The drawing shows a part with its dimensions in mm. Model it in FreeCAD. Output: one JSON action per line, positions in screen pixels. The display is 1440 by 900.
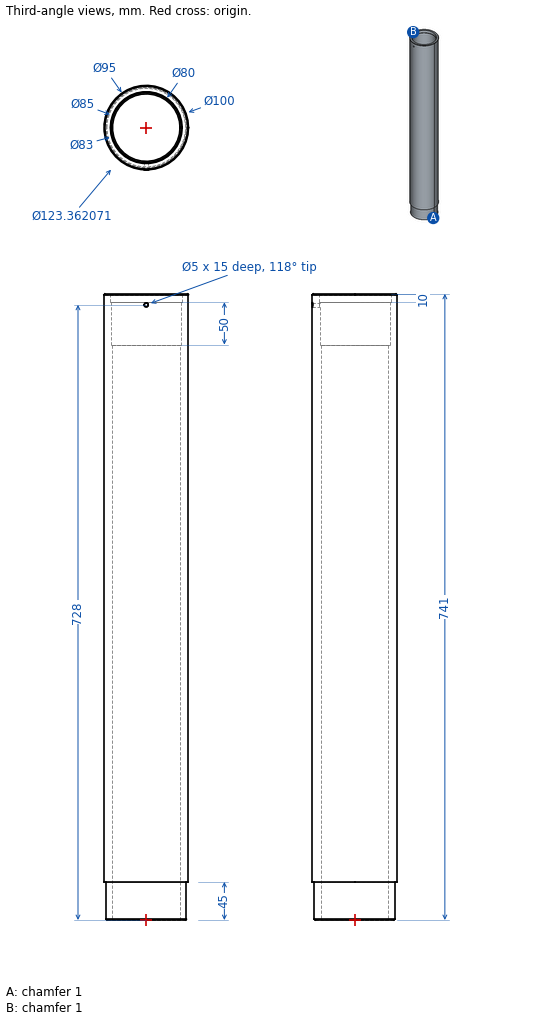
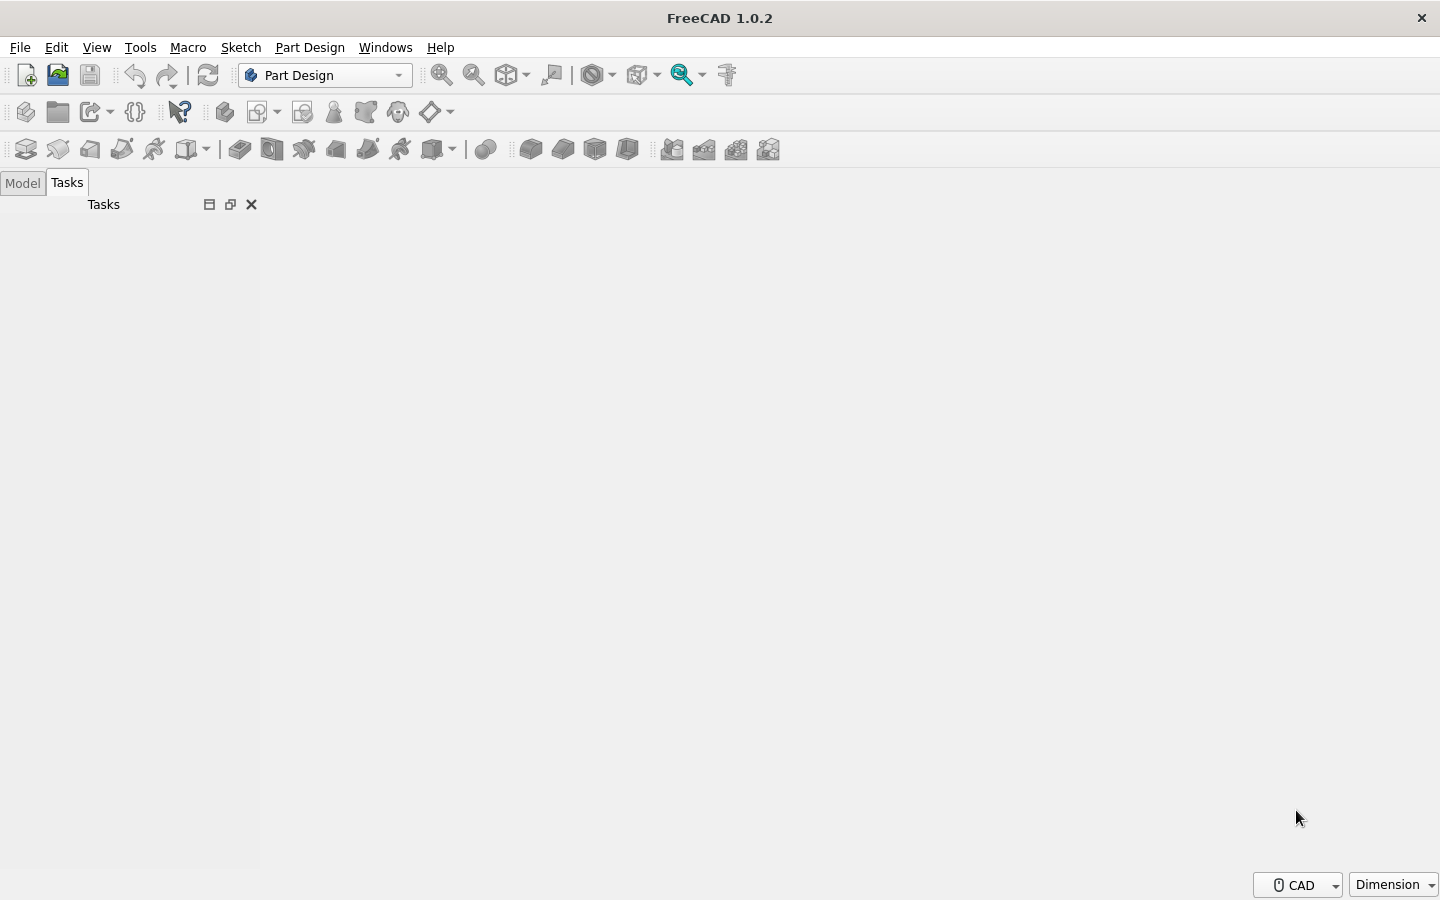
{"action": "left_click", "coordinate": [26, 76]}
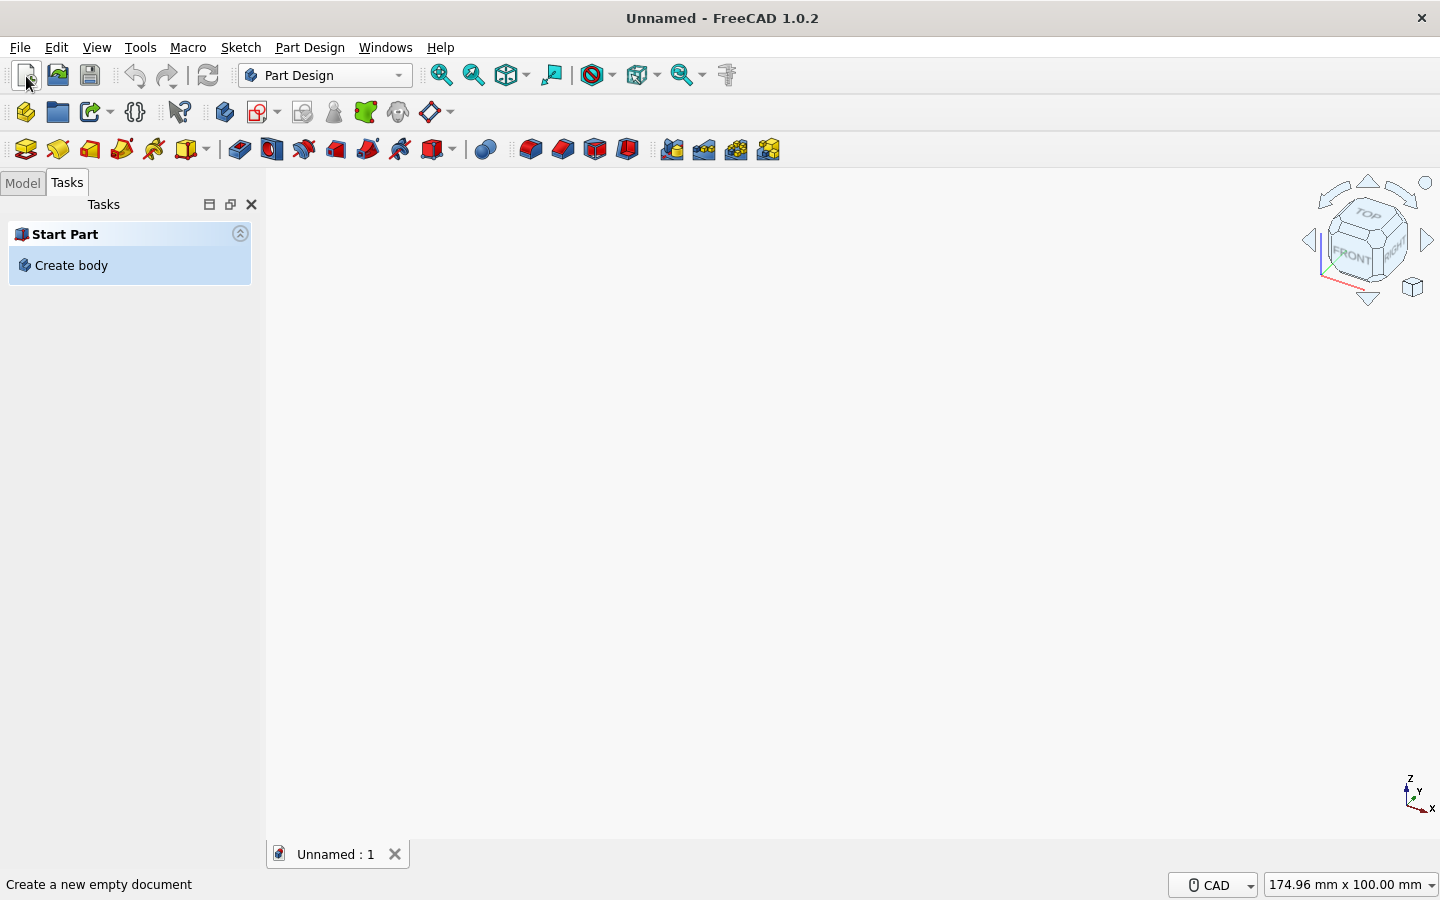
{"action": "left_click", "coordinate": [258, 112]}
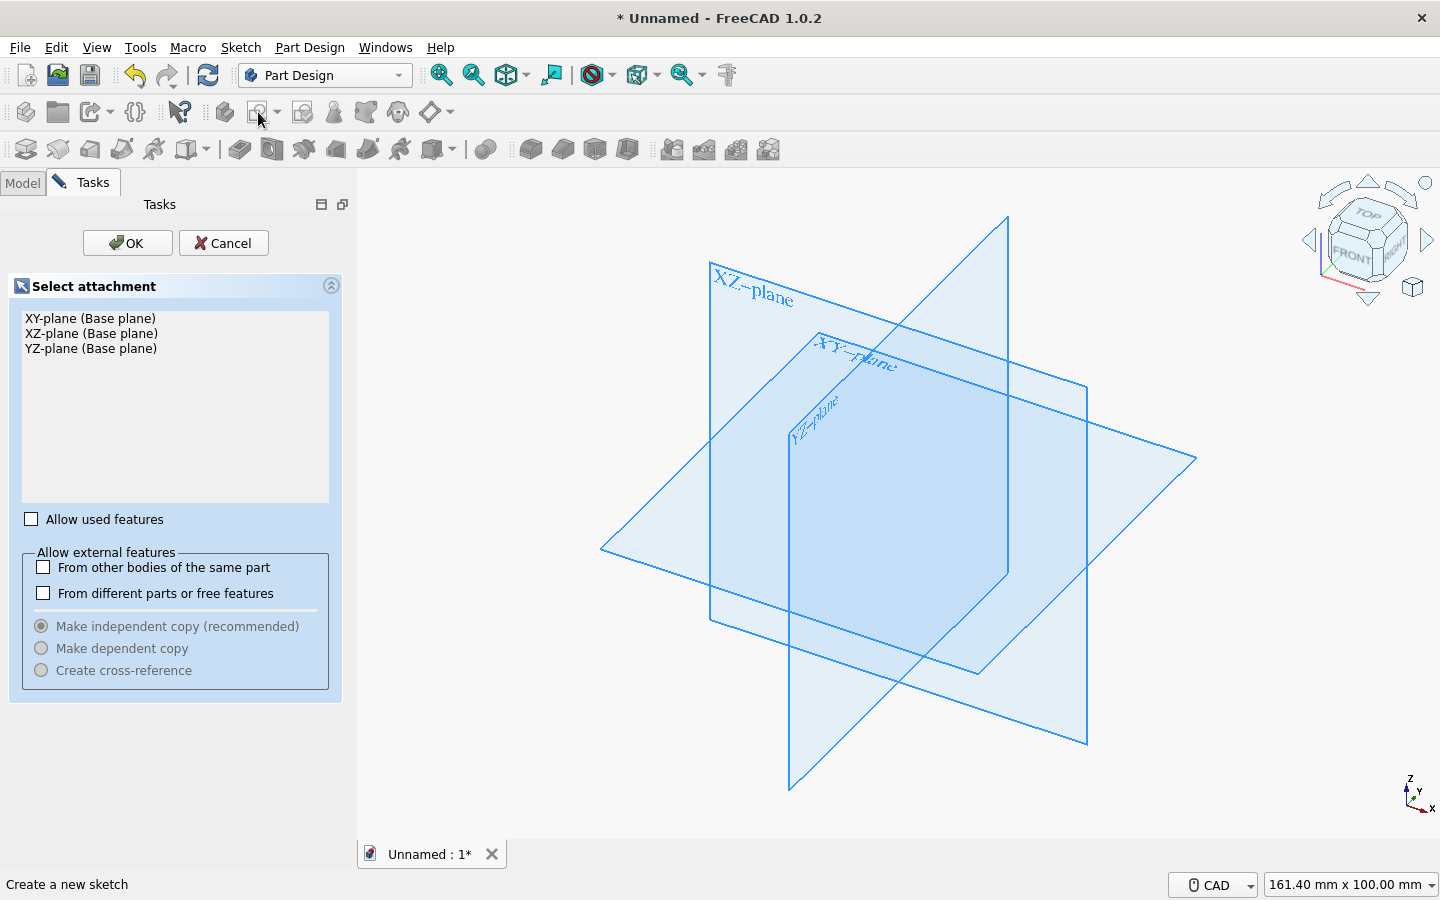
{"action": "left_click", "coordinate": [82, 318]}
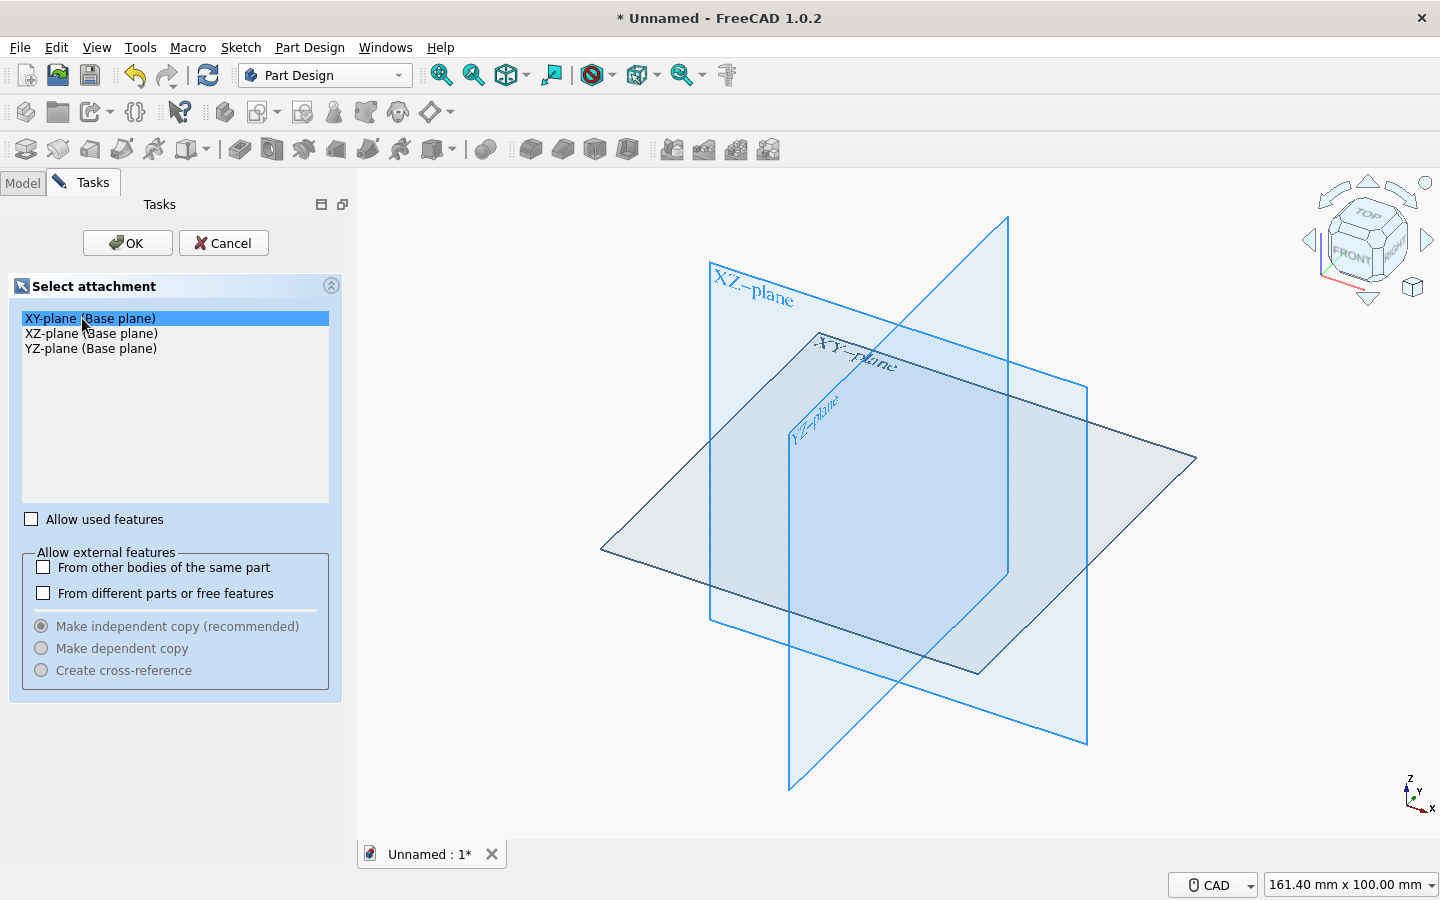
{"action": "left_click", "coordinate": [128, 243]}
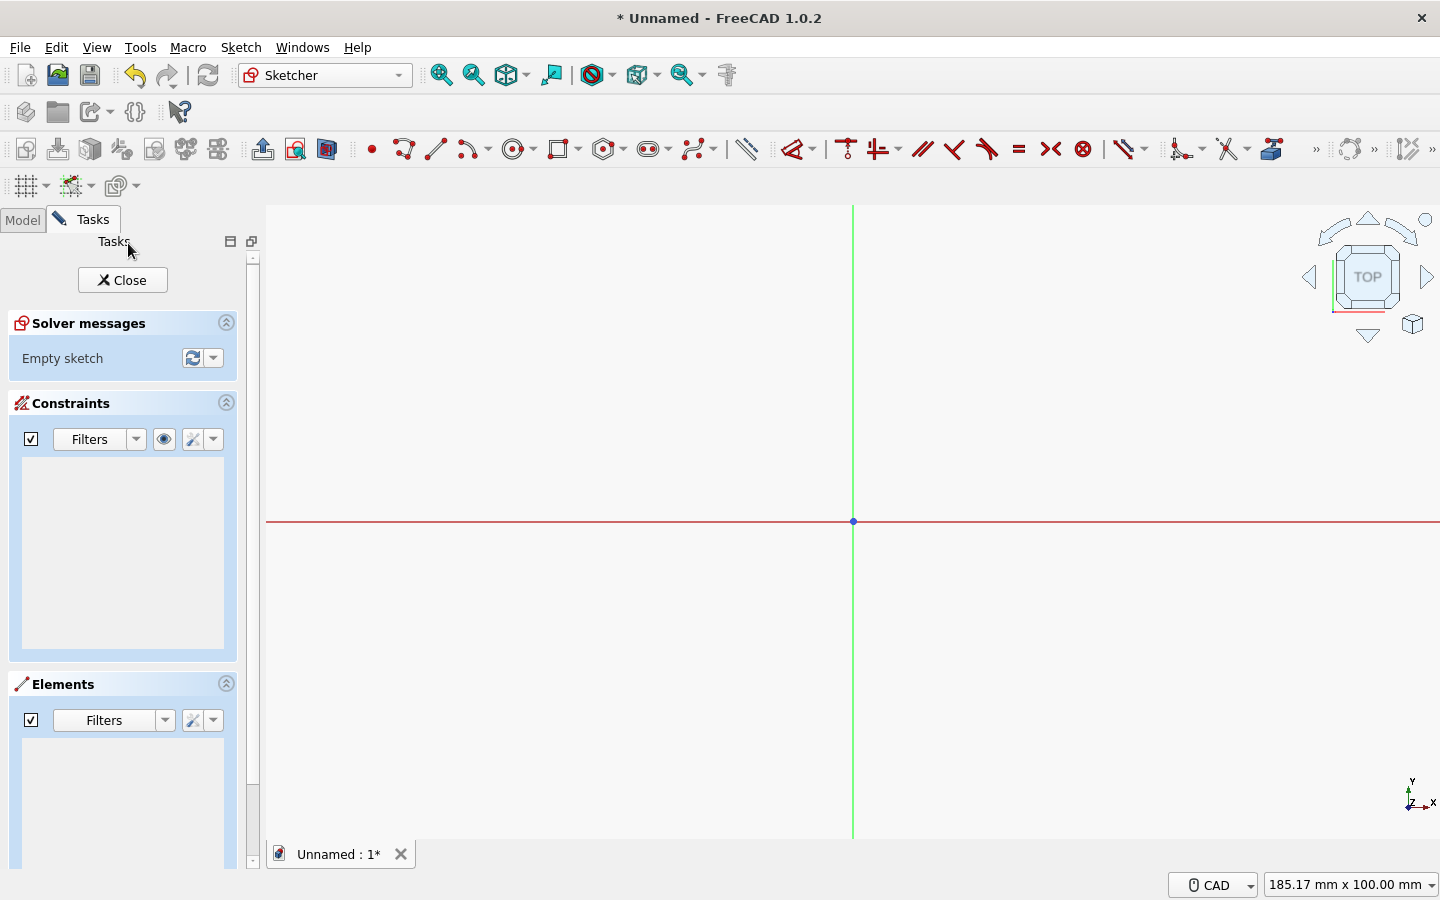
{"action": "scroll", "coordinate": [645, 522], "scroll_direction": "down", "scroll_amount": 2}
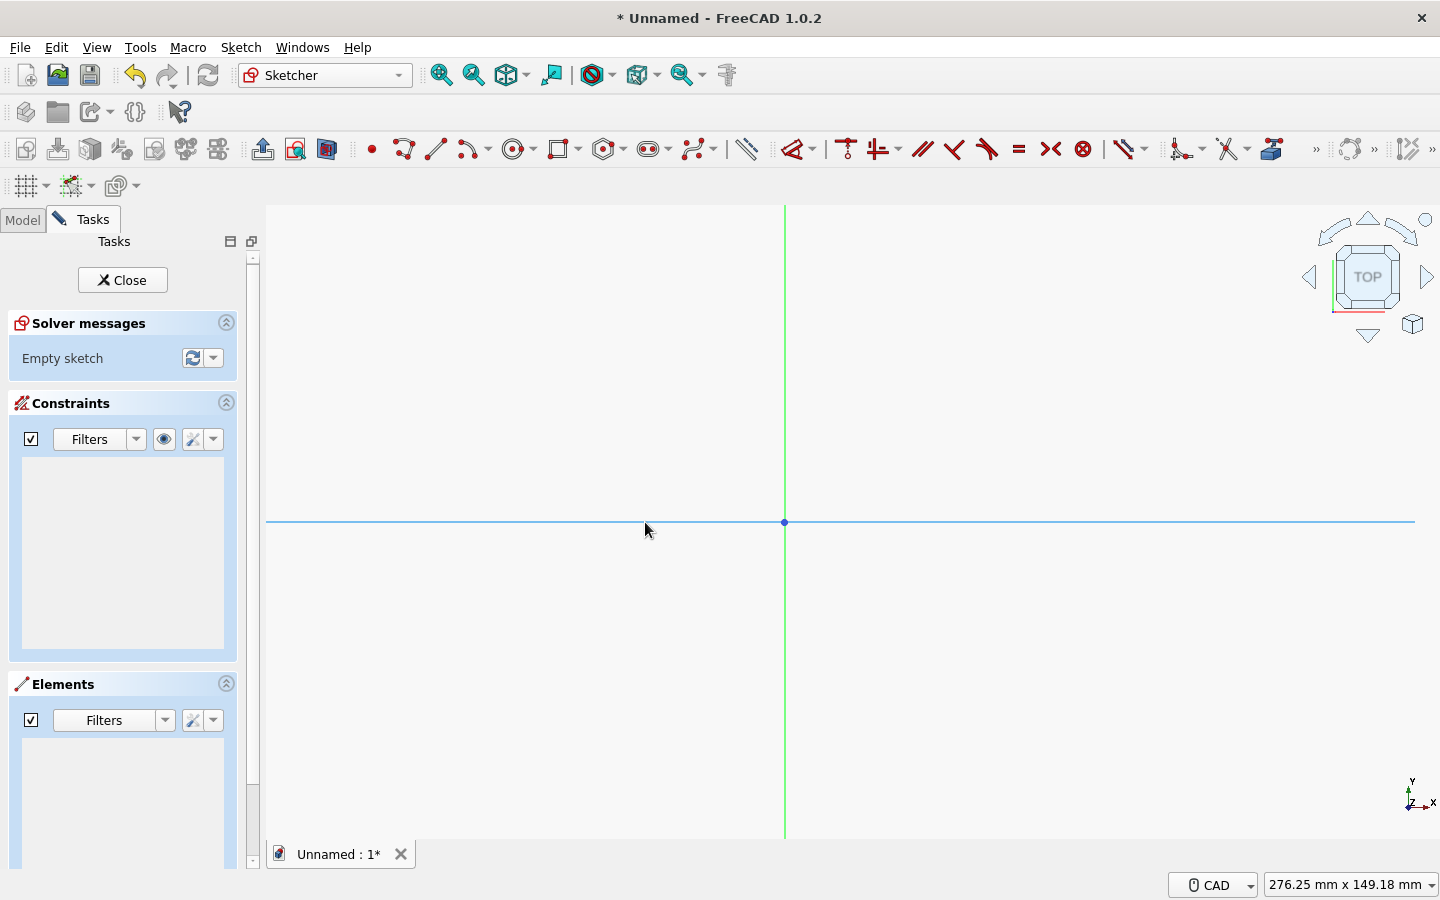
{"action": "left_click", "coordinate": [514, 150]}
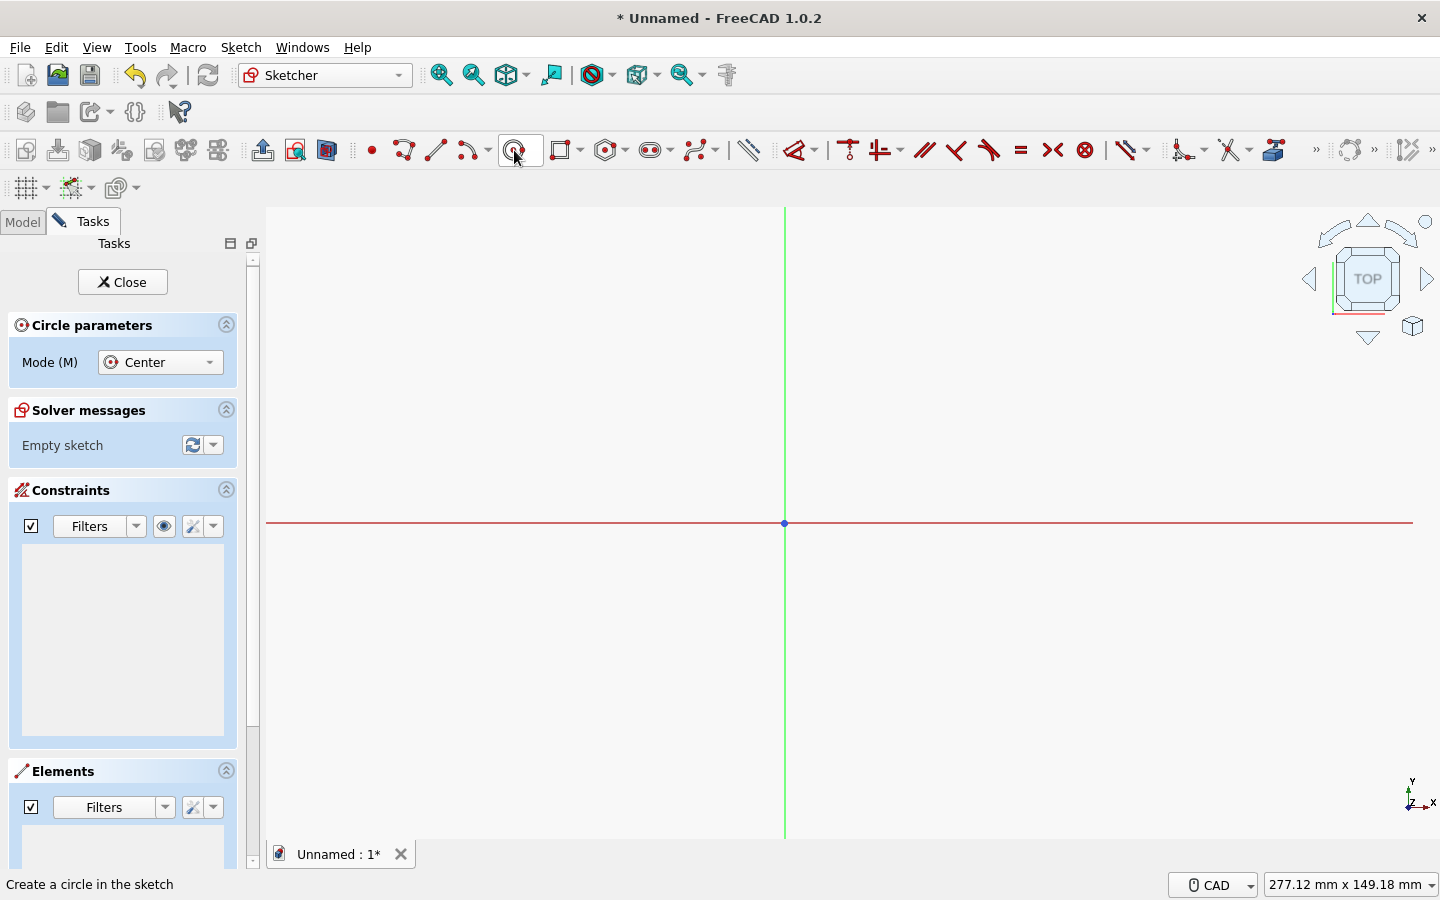
{"action": "left_click", "coordinate": [785, 523]}
{"action": "left_click", "coordinate": [935, 373]}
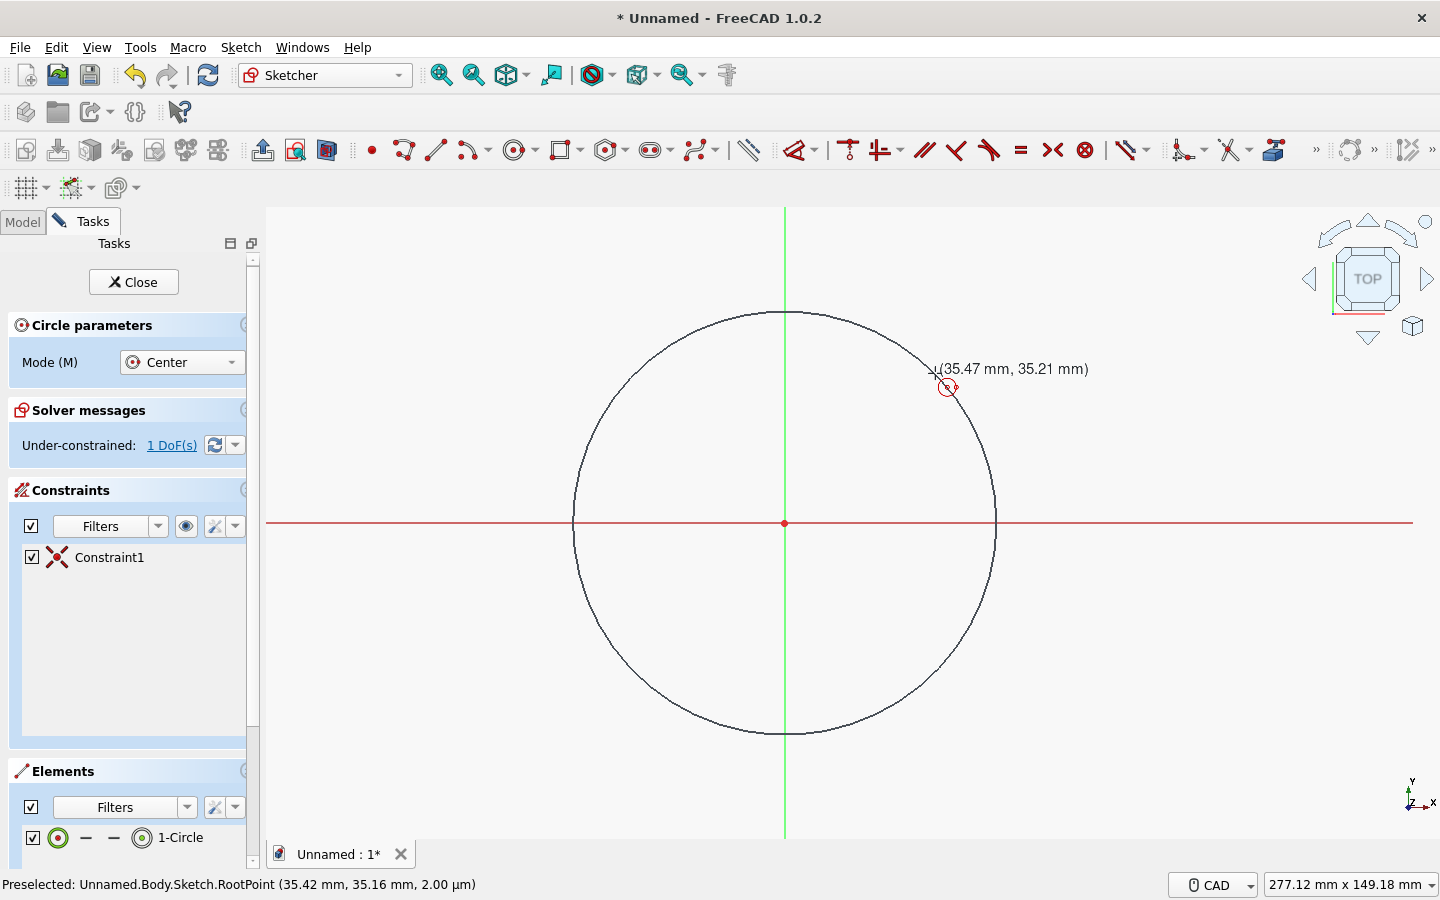
{"action": "left_click", "coordinate": [785, 523]}
{"action": "left_click", "coordinate": [905, 403]}
{"action": "key", "text": "Escape"}